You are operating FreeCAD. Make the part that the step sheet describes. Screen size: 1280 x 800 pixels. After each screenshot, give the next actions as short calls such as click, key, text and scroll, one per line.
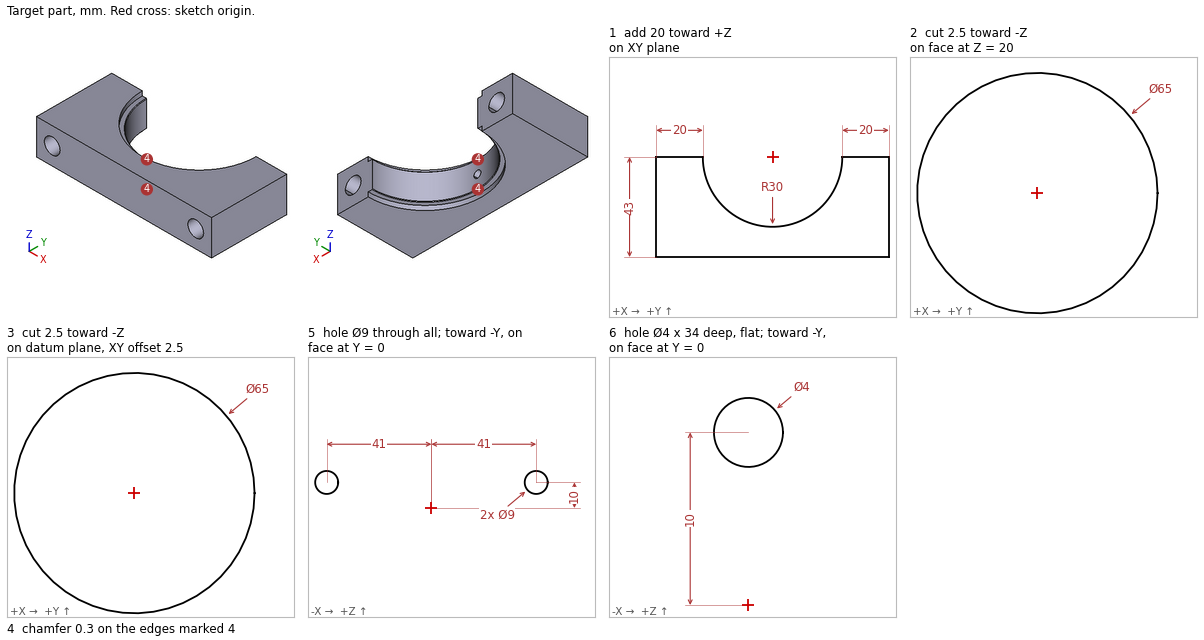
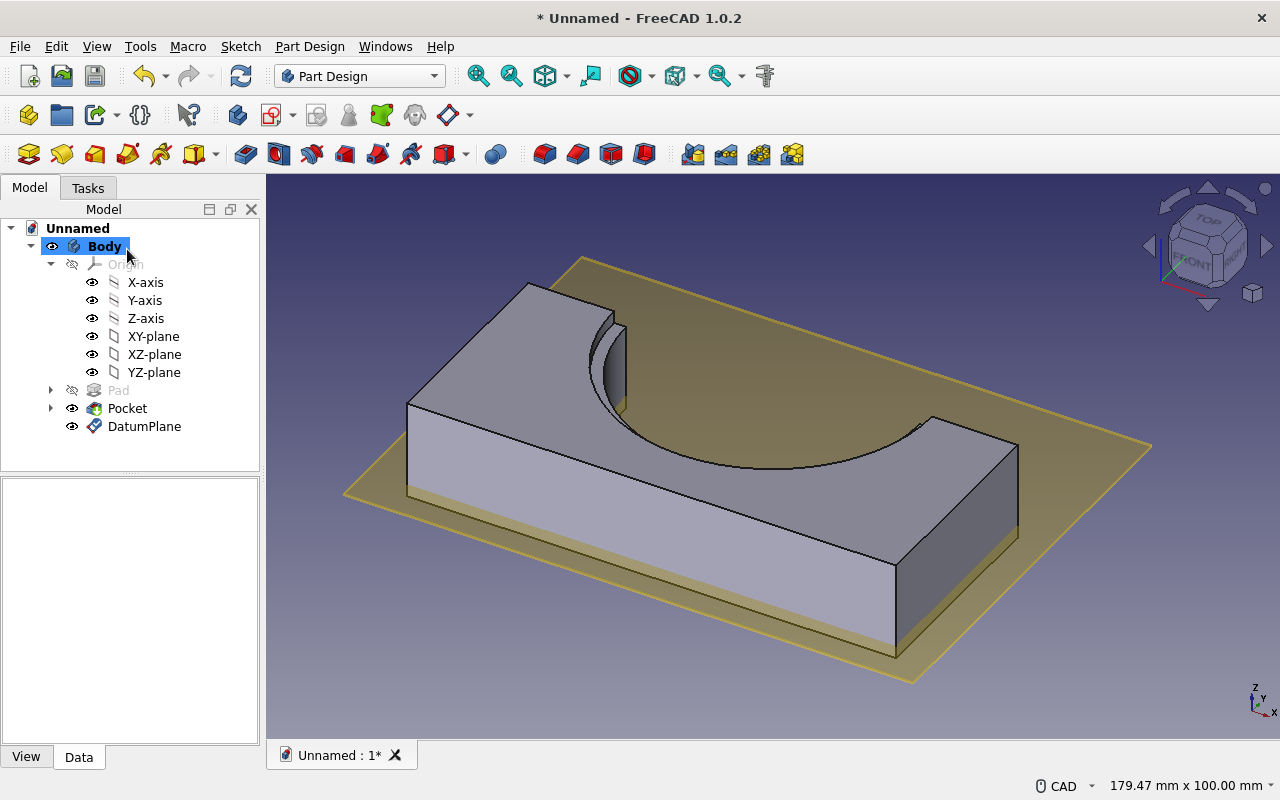
click(117, 426)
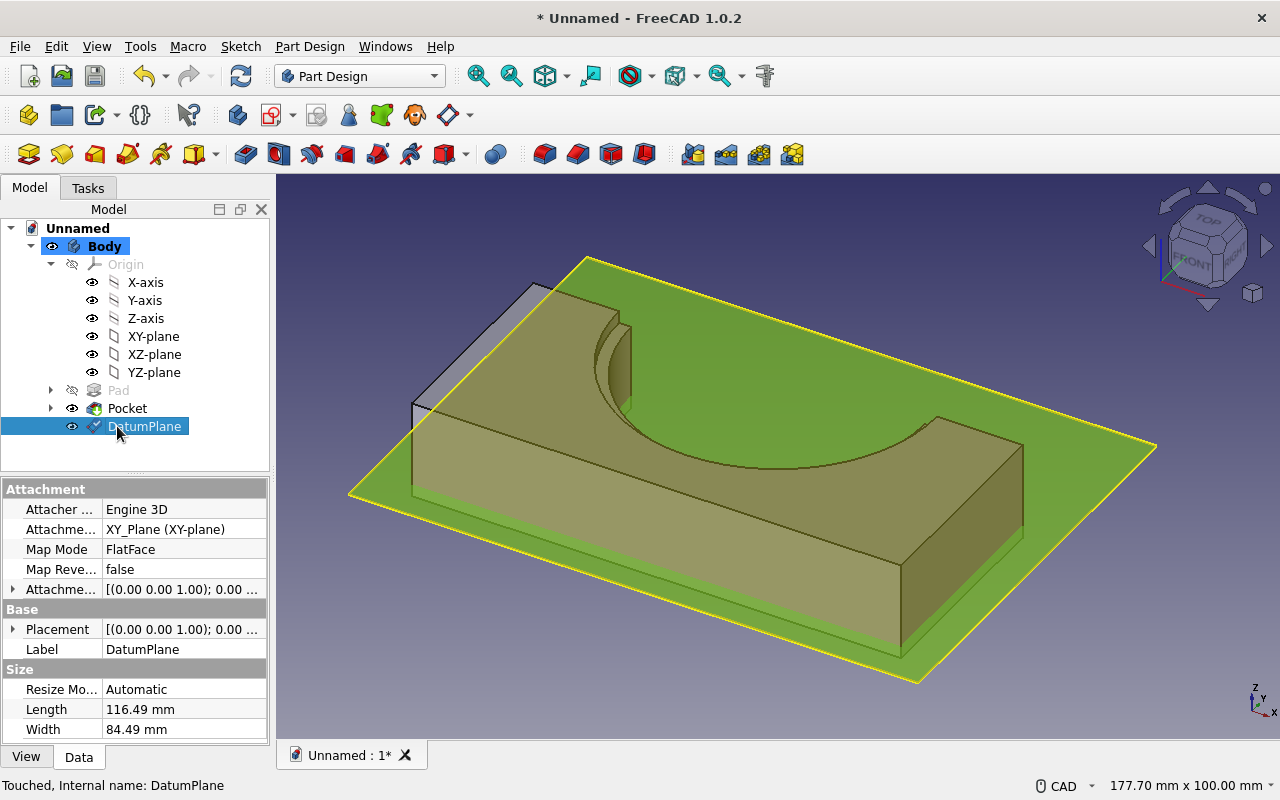
click(270, 116)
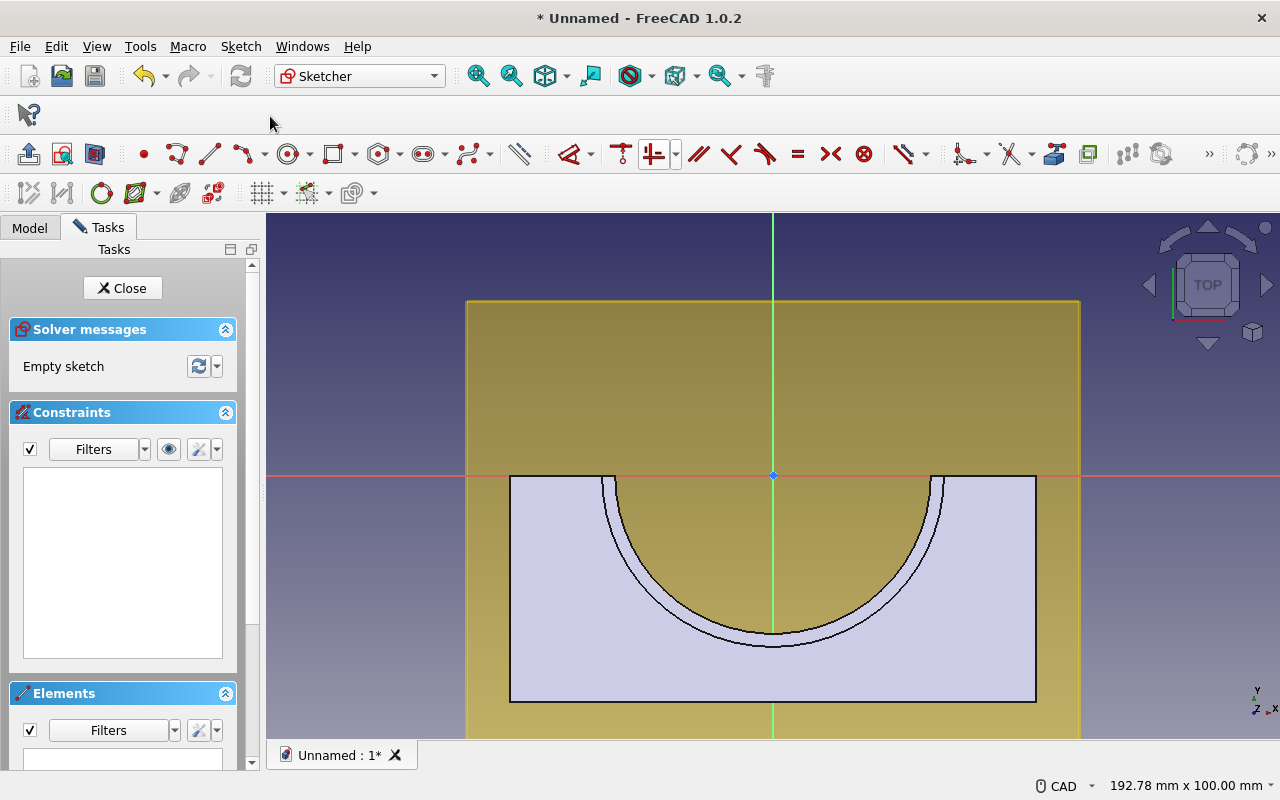
click(95, 154)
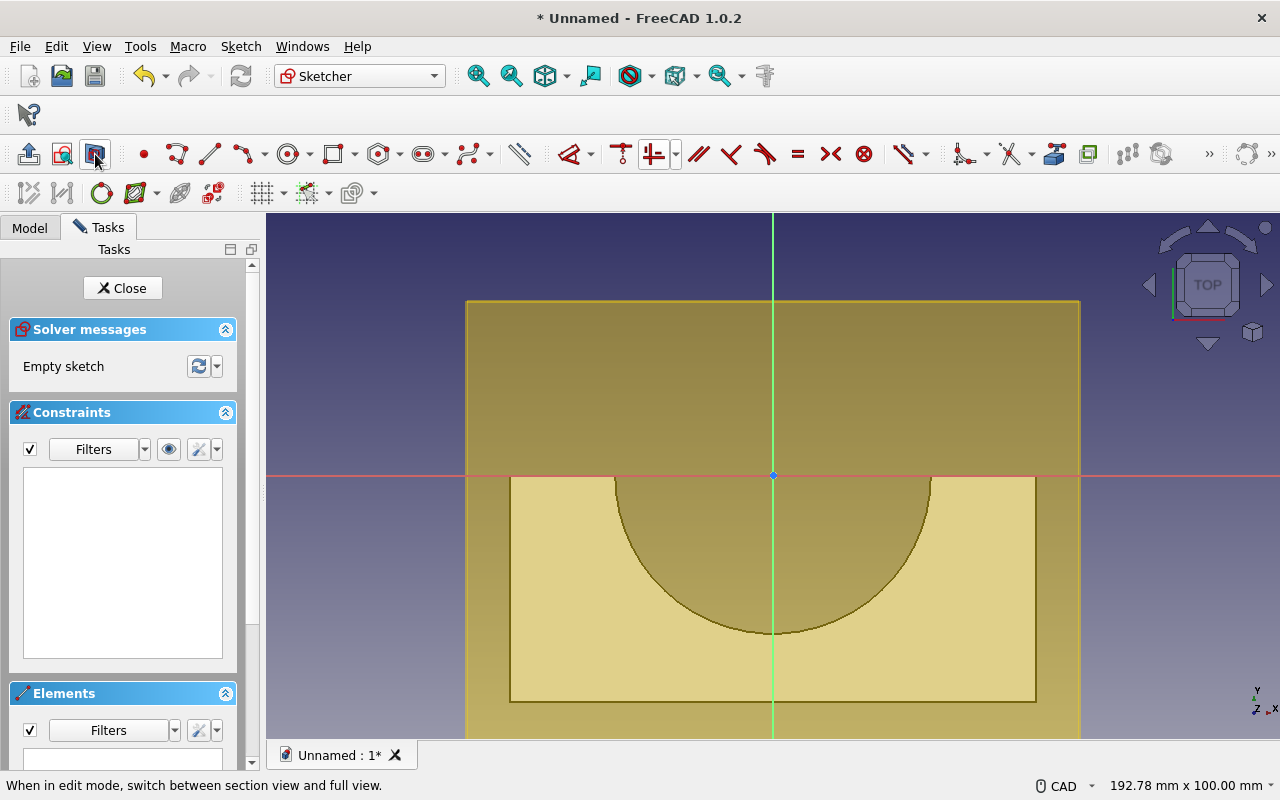
click(288, 154)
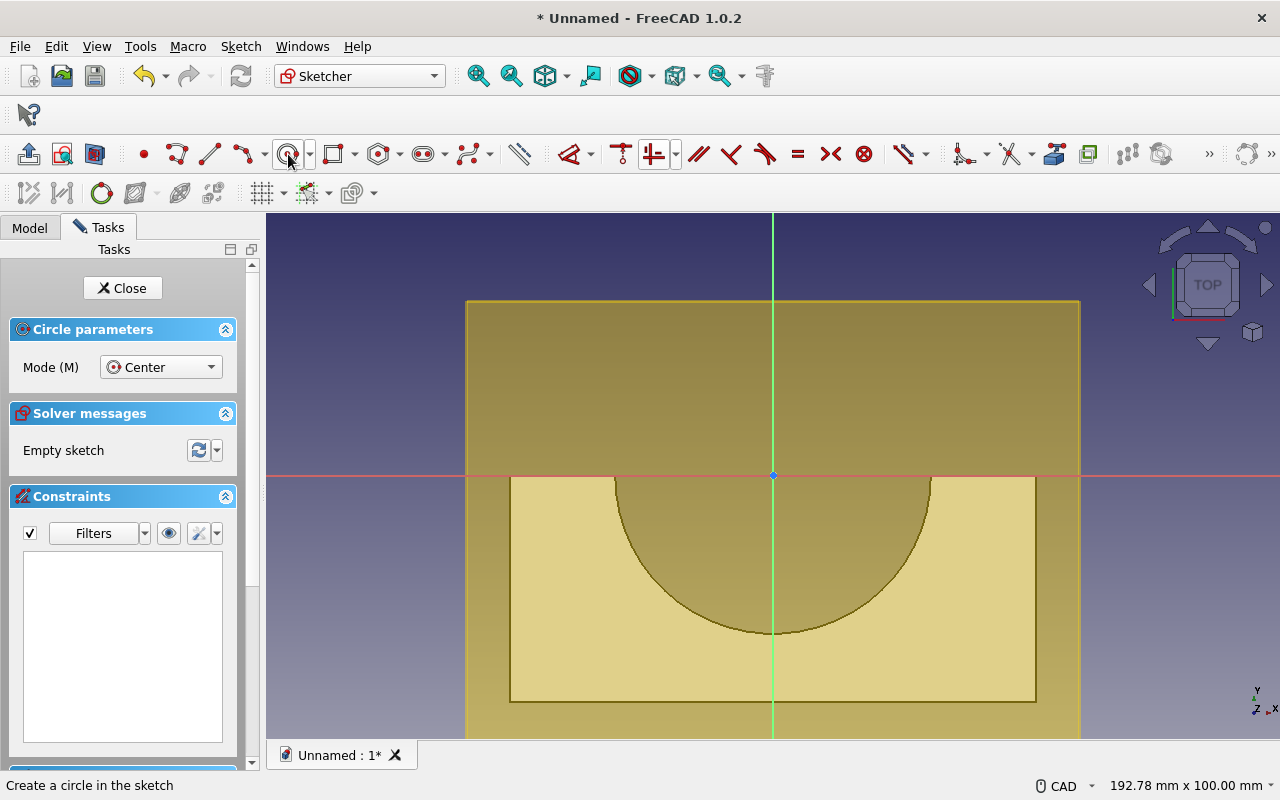
click(773, 476)
click(894, 355)
key(Escape)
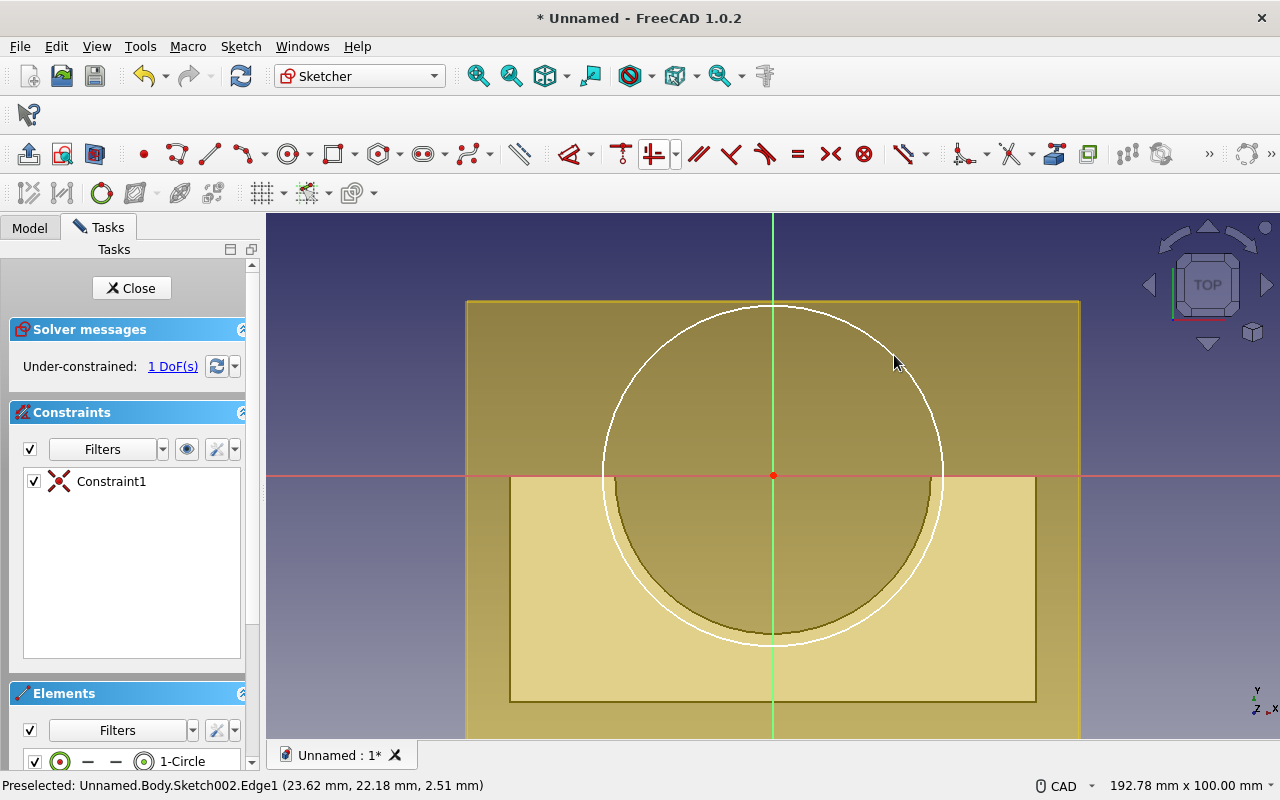
click(568, 154)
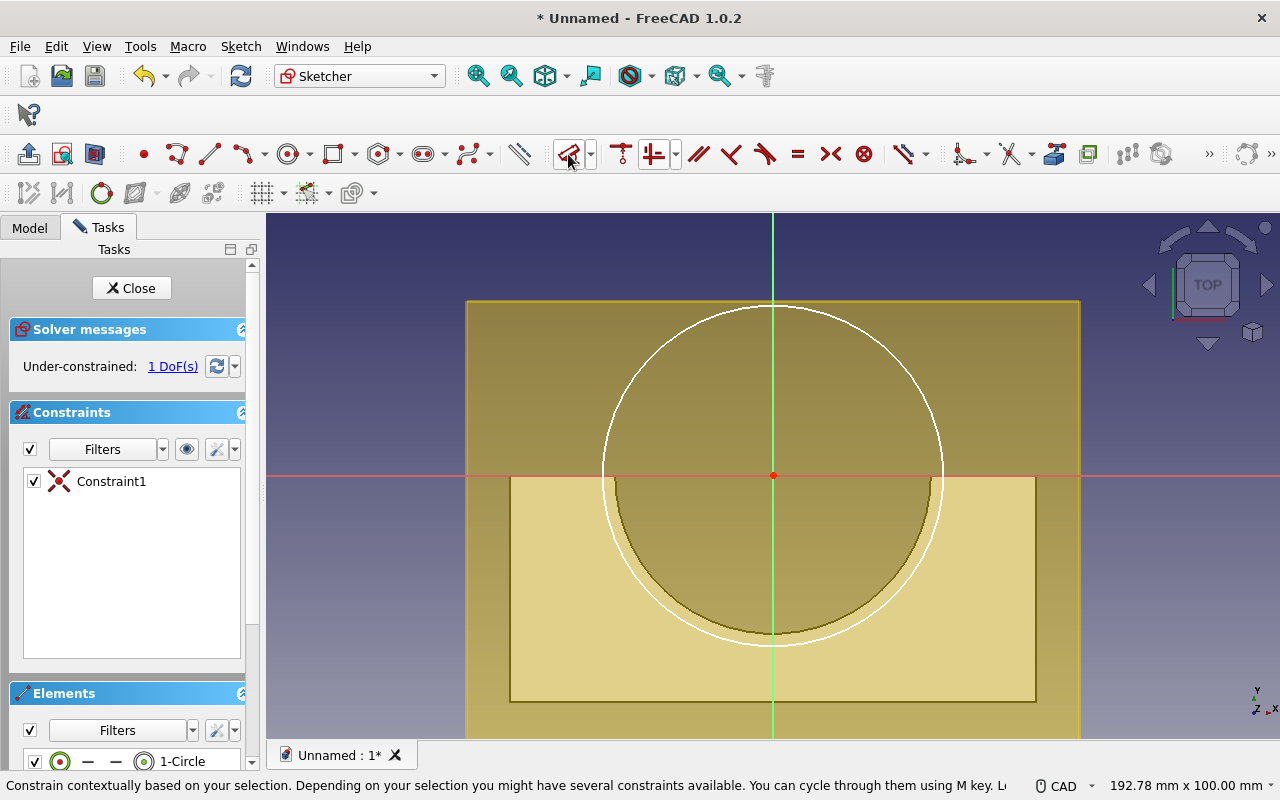
click(893, 355)
click(916, 332)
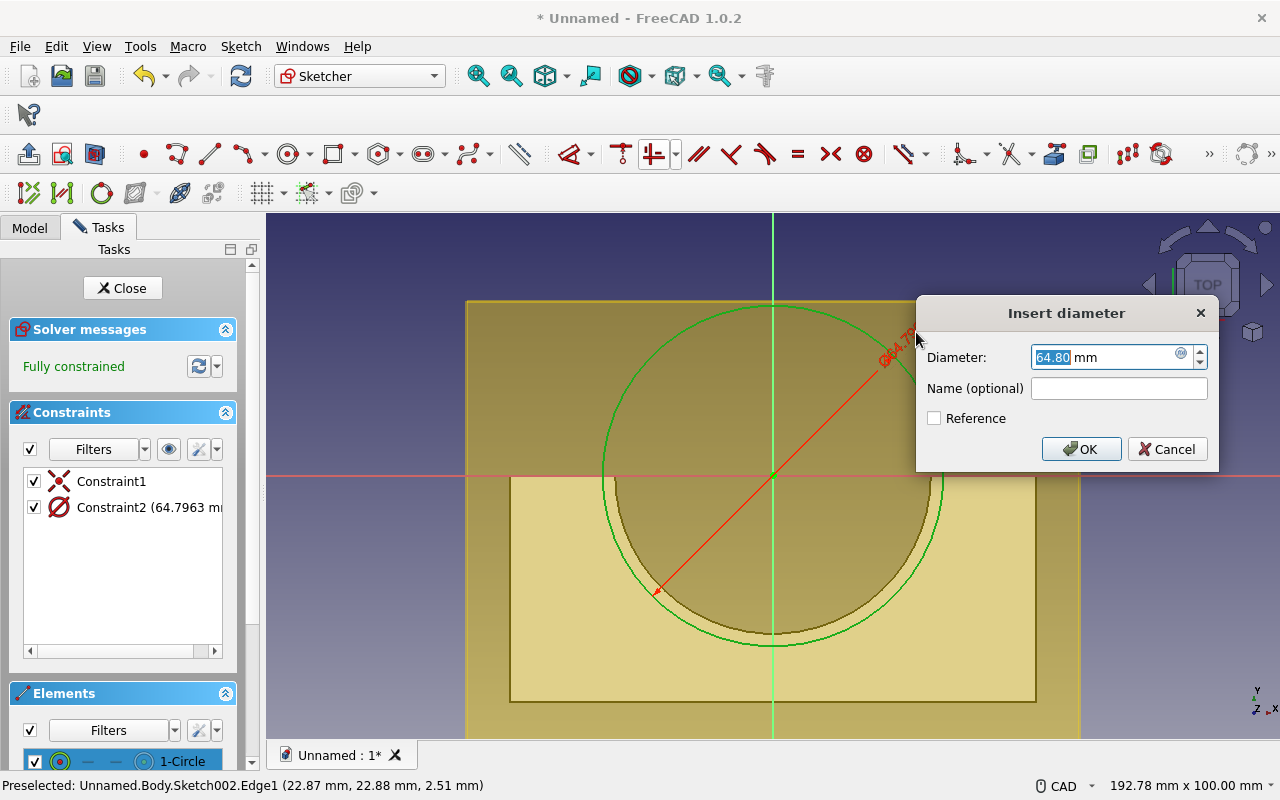
text(65)
key(Return)
key(Escape)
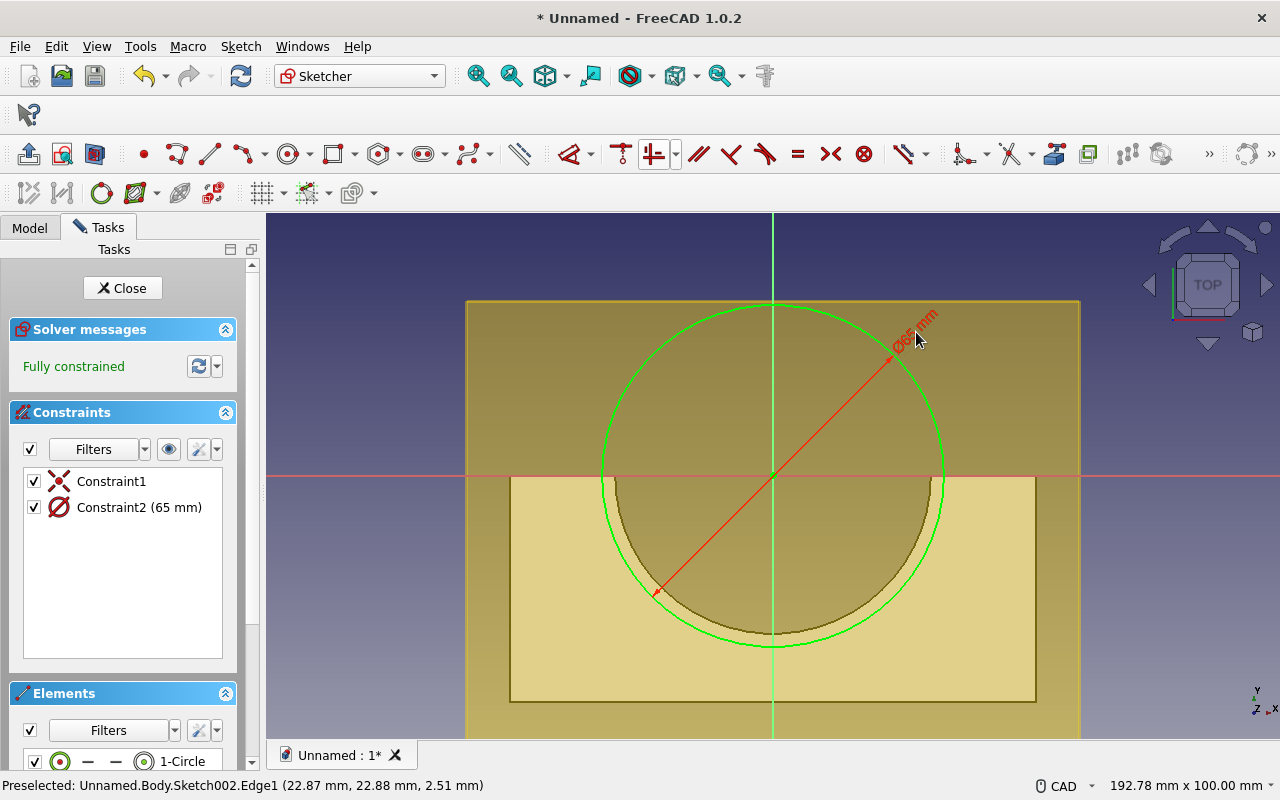
click(123, 288)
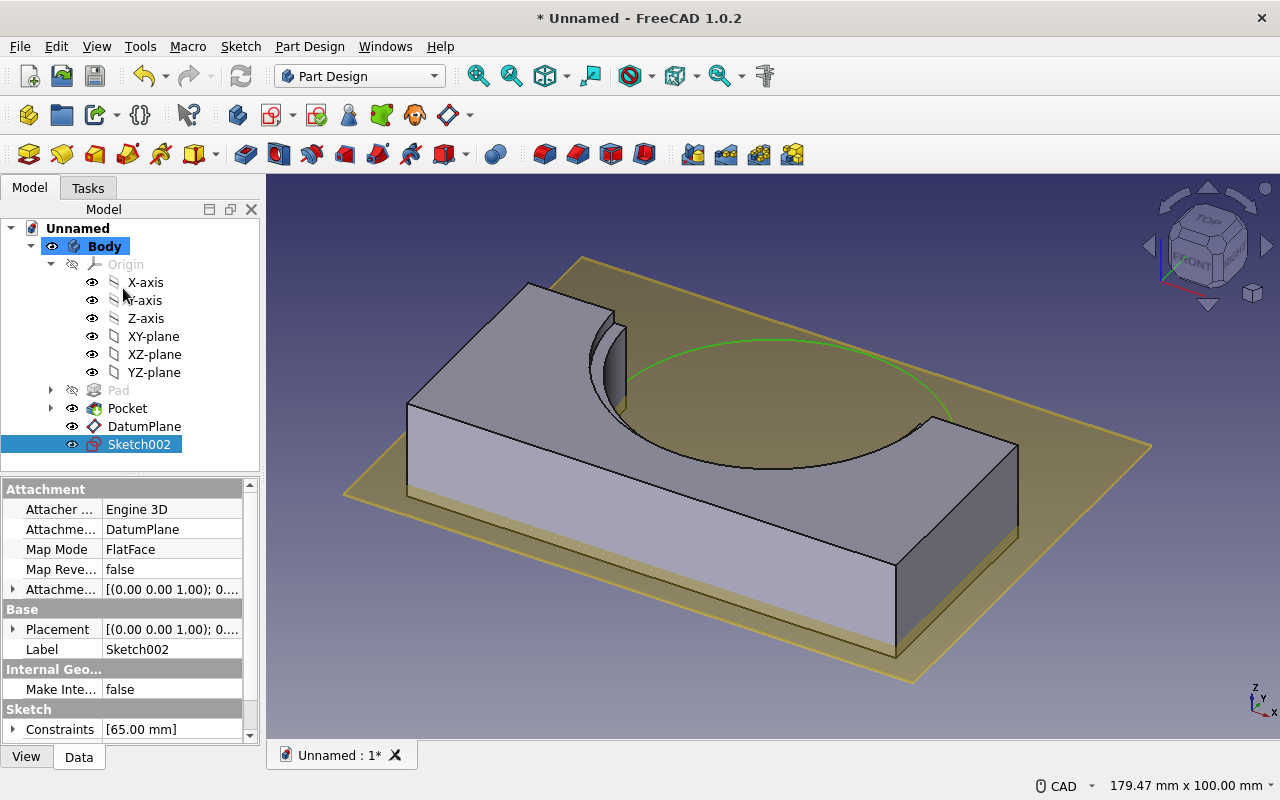
click(246, 154)